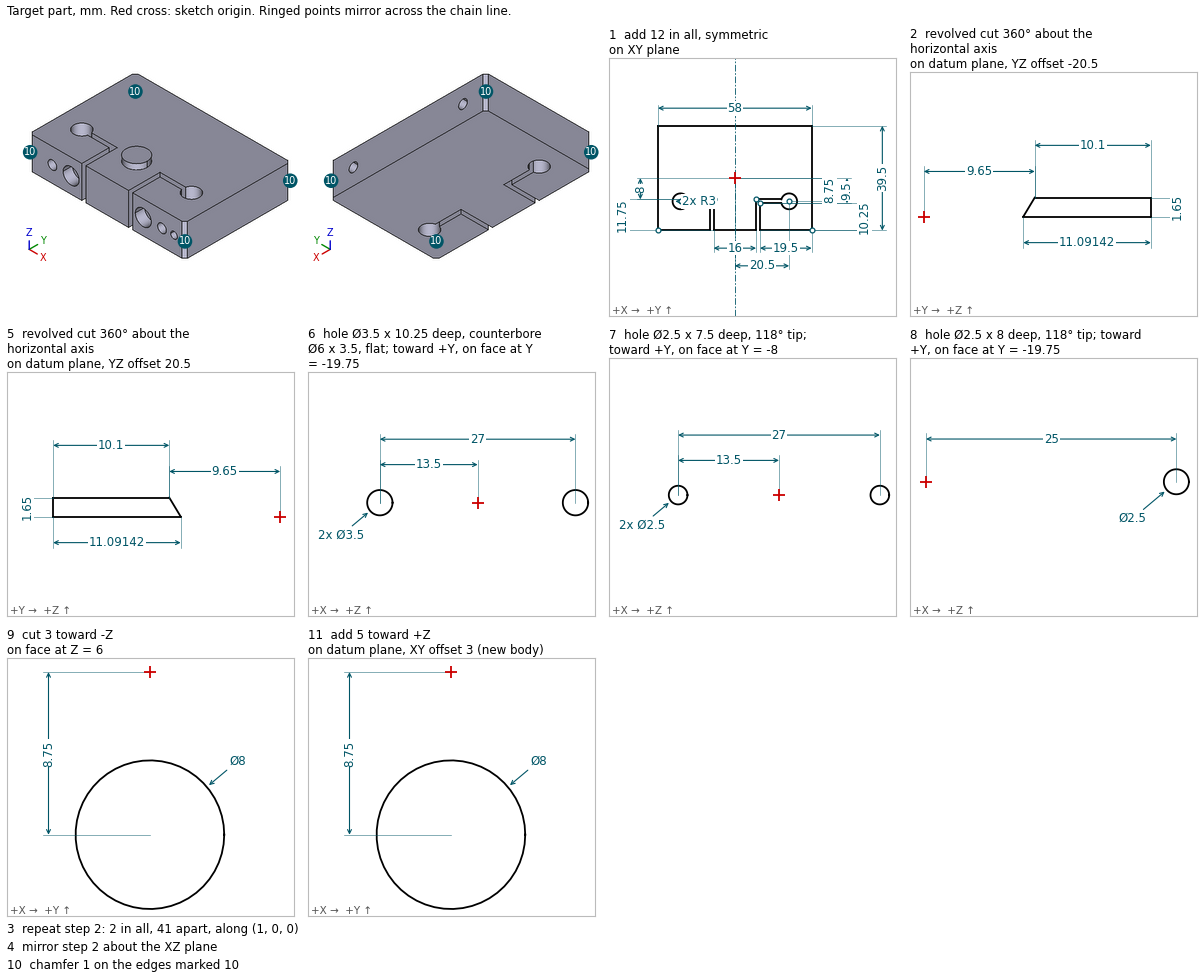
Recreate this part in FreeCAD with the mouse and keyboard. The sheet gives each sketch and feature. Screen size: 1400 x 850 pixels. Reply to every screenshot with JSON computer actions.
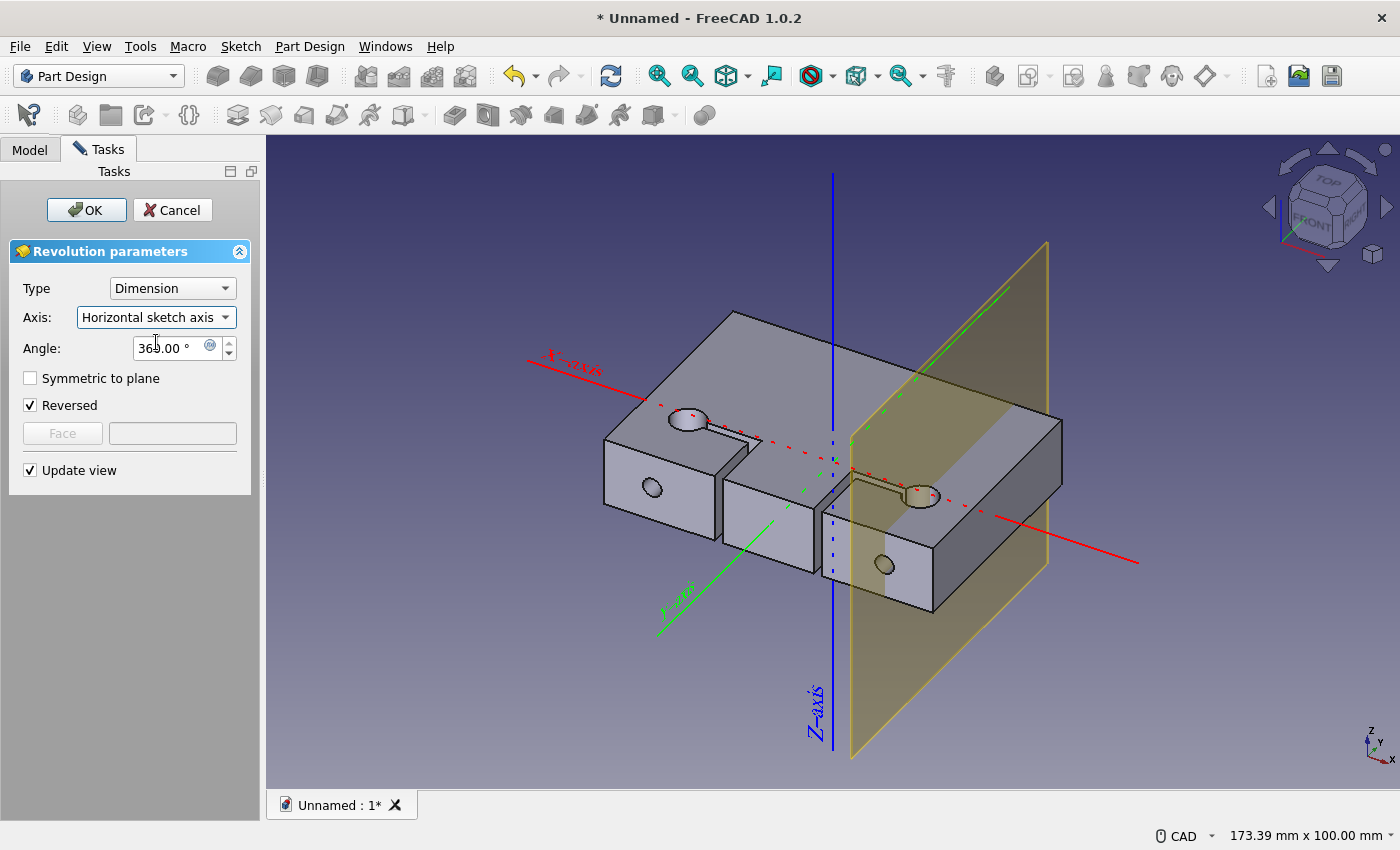
{"action": "left_click", "coordinate": [87, 210]}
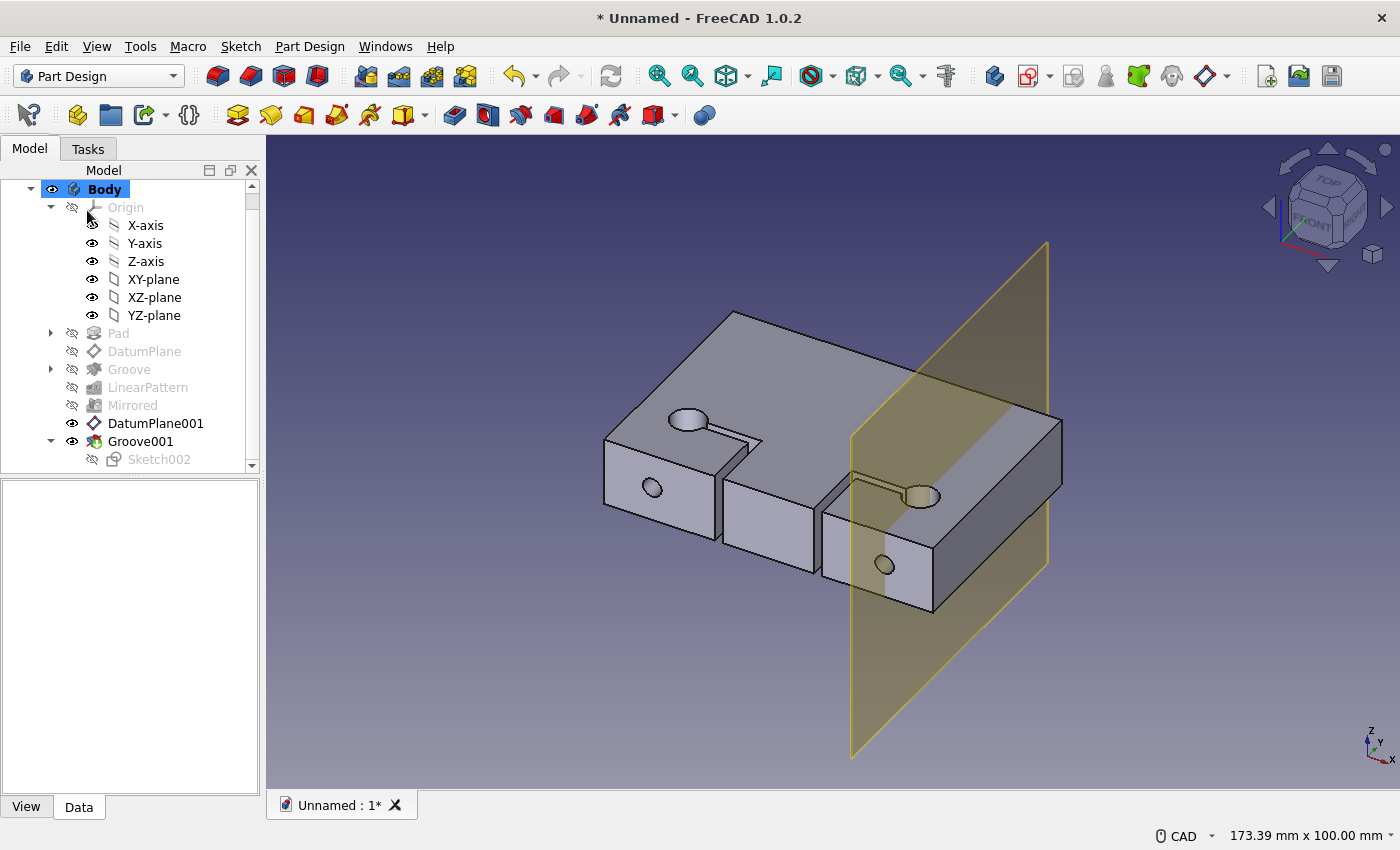
{"action": "left_click", "coordinate": [117, 423]}
{"action": "key", "text": "space"}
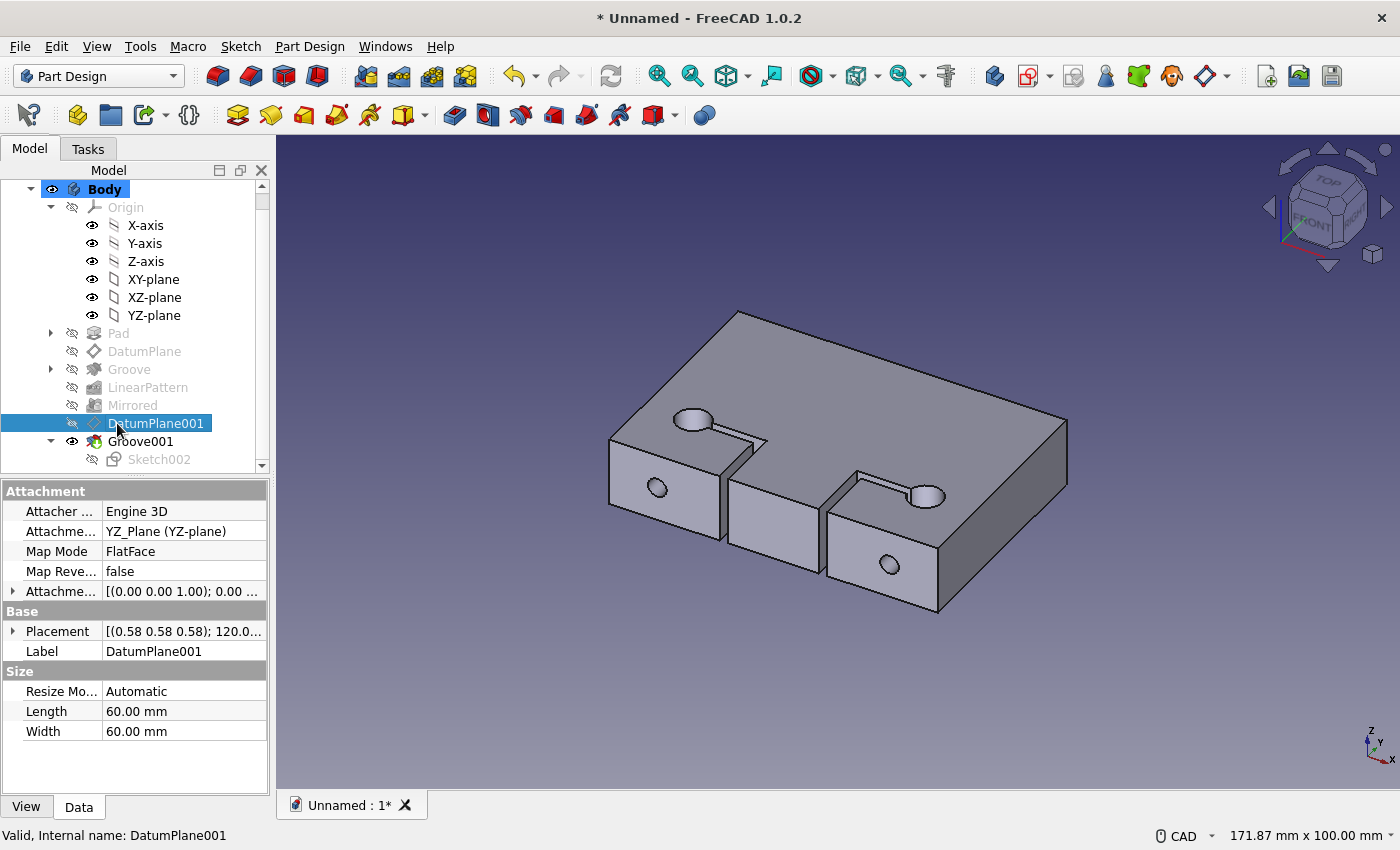
{"action": "left_click", "coordinate": [696, 490]}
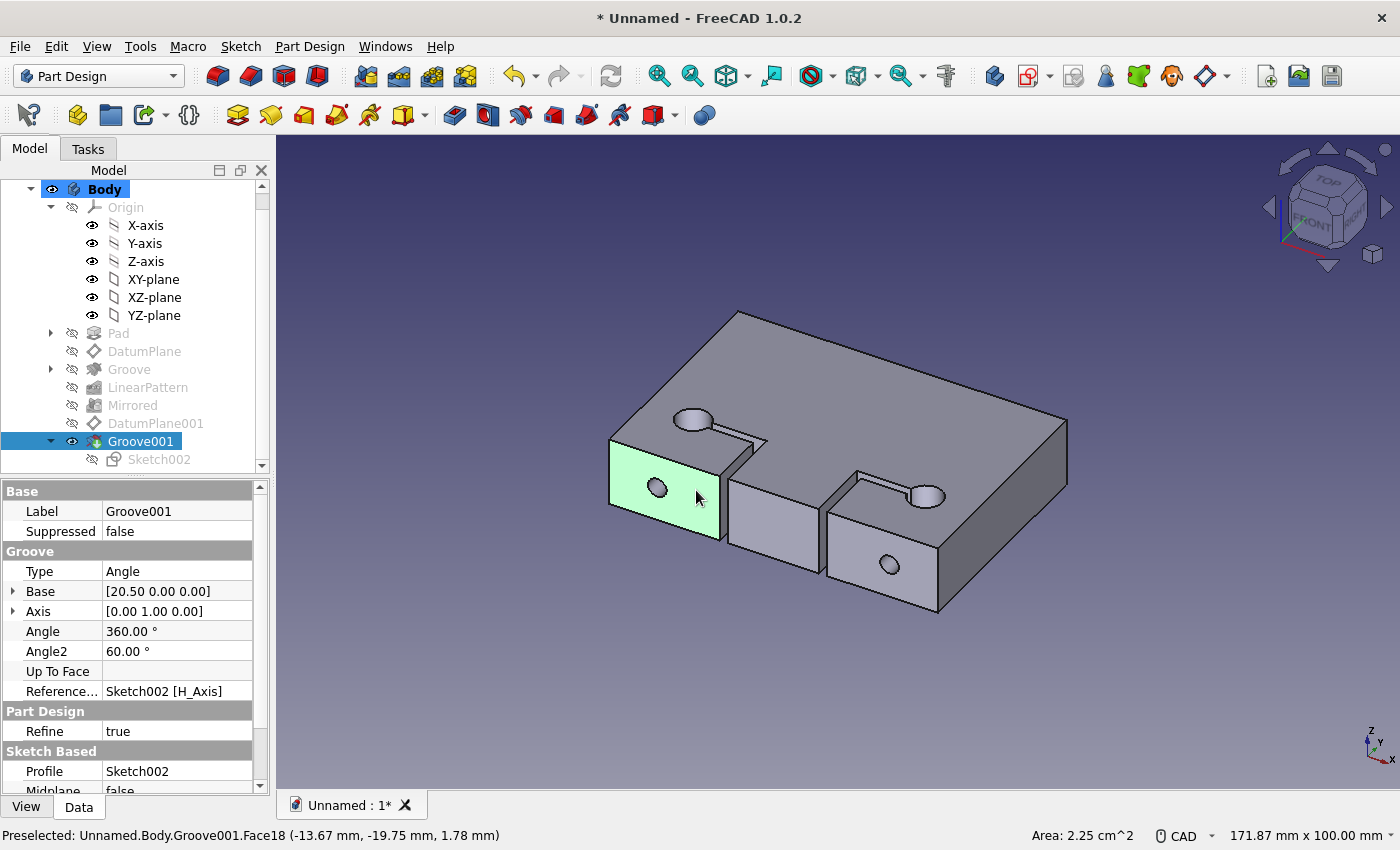
{"action": "left_click", "coordinate": [1028, 76]}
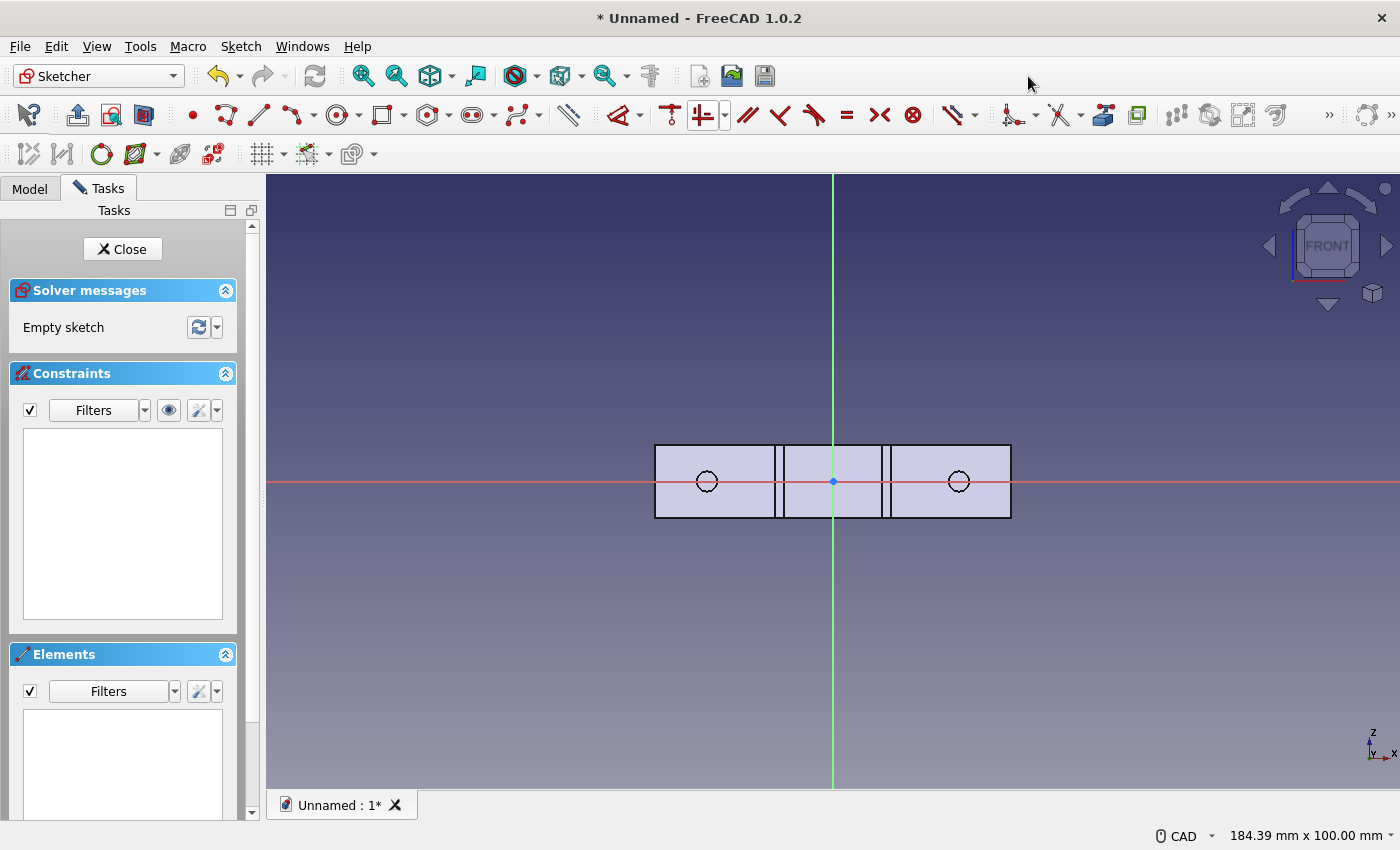
{"action": "scroll", "coordinate": [863, 482], "scroll_direction": "up", "scroll_amount": 6}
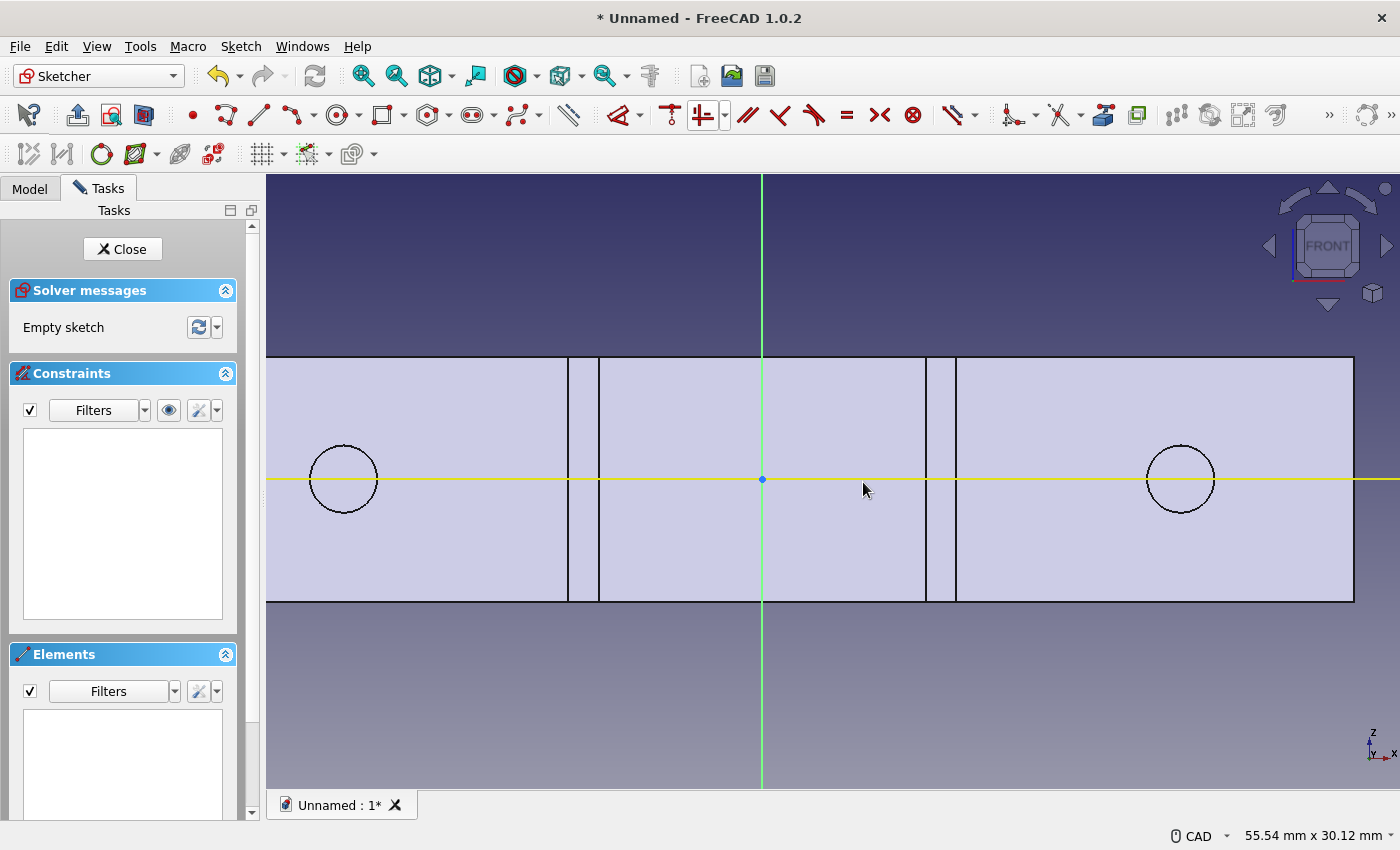
{"action": "left_click", "coordinate": [336, 116]}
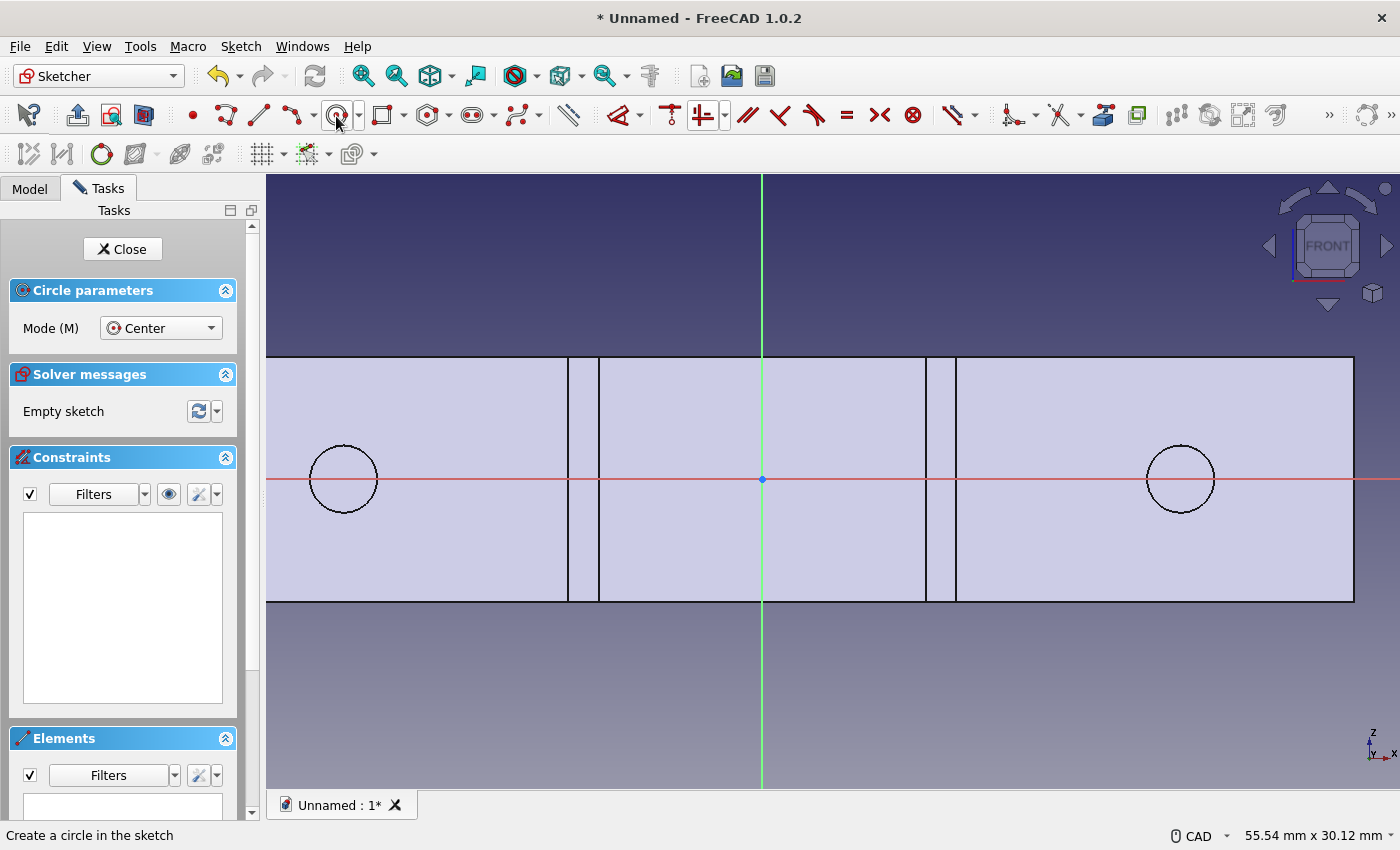
{"action": "left_click", "coordinate": [487, 479]}
{"action": "left_click", "coordinate": [512, 454]}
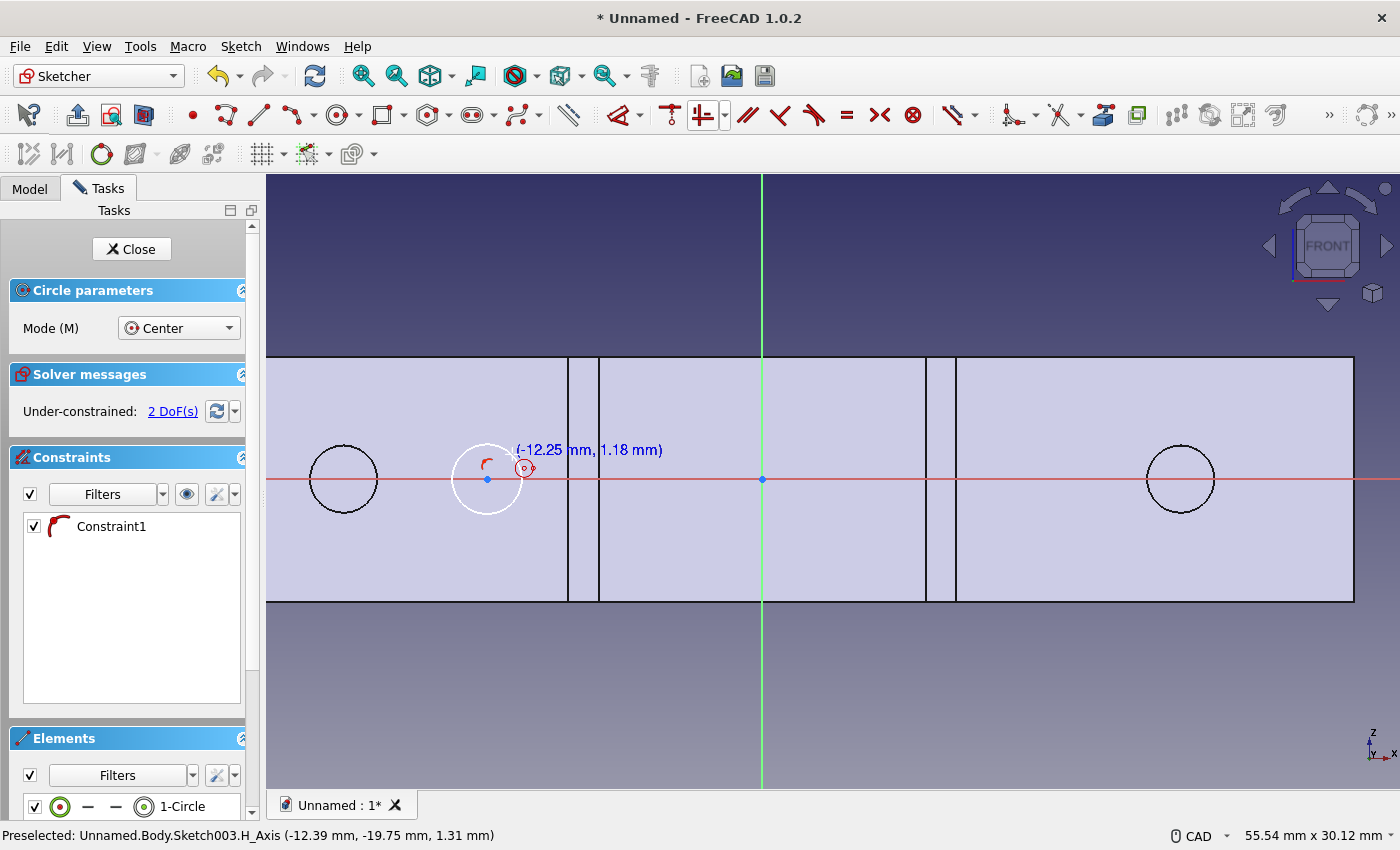
{"action": "left_click", "coordinate": [1038, 479]}
{"action": "left_click", "coordinate": [1063, 454]}
{"action": "key", "text": "Escape"}